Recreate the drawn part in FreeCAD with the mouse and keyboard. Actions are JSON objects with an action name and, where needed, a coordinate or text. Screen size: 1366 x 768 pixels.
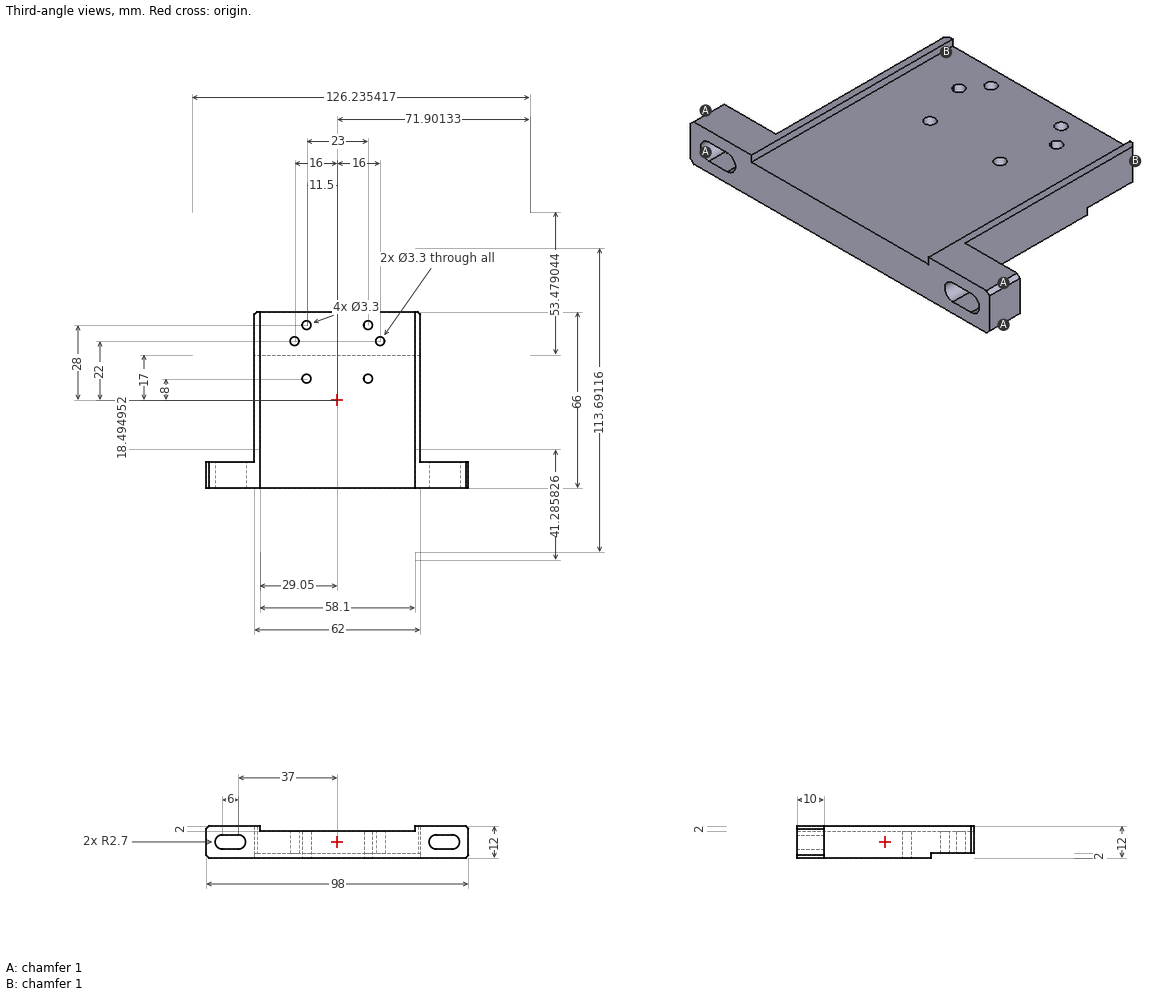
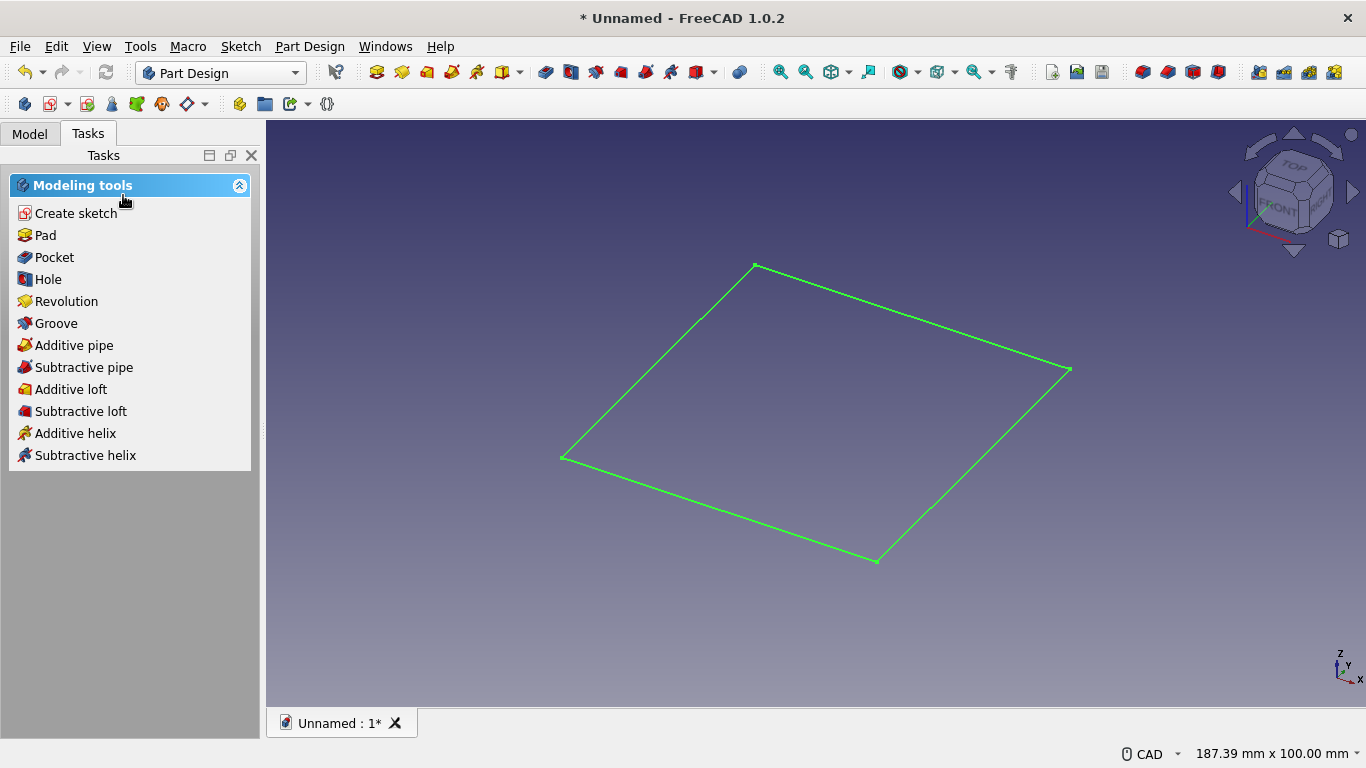
{"action": "left_click", "coordinate": [377, 72]}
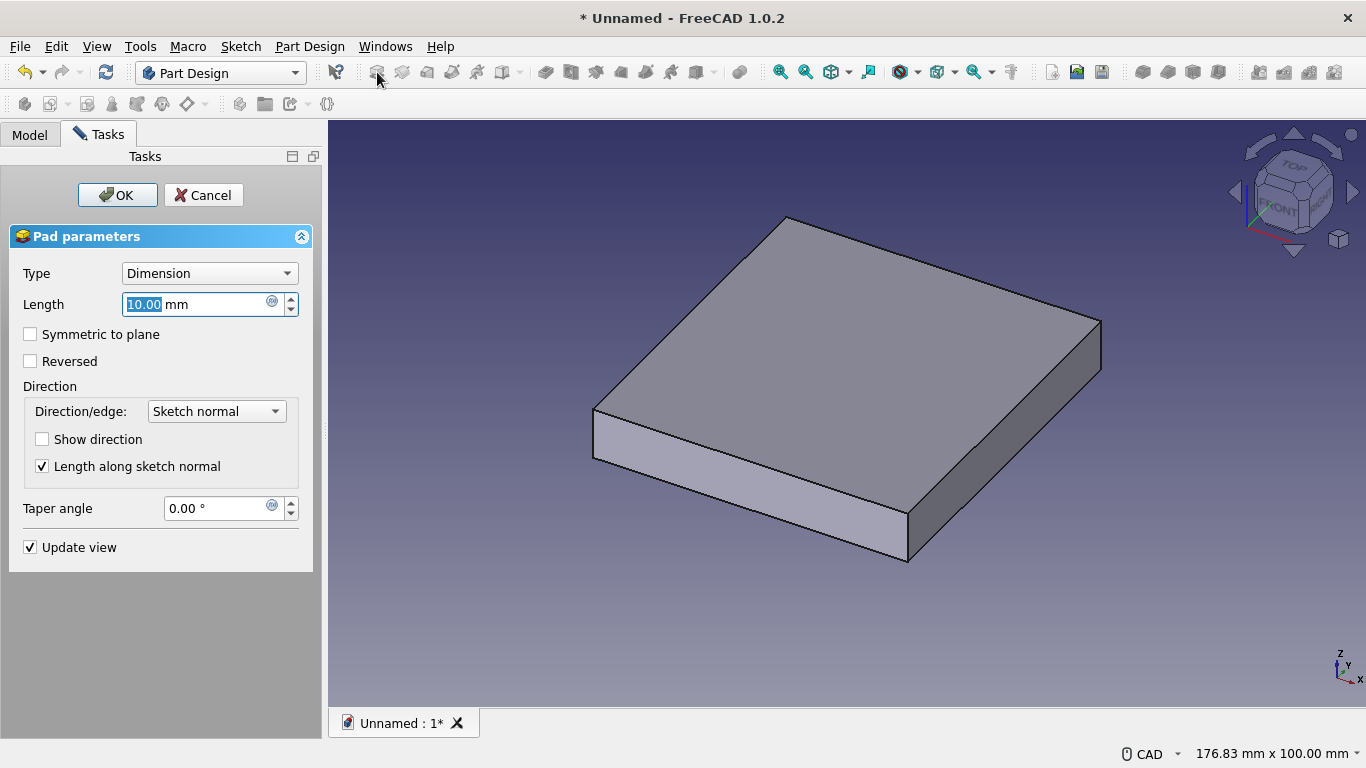
{"action": "type", "text": "12"}
{"action": "key", "text": "Tab"}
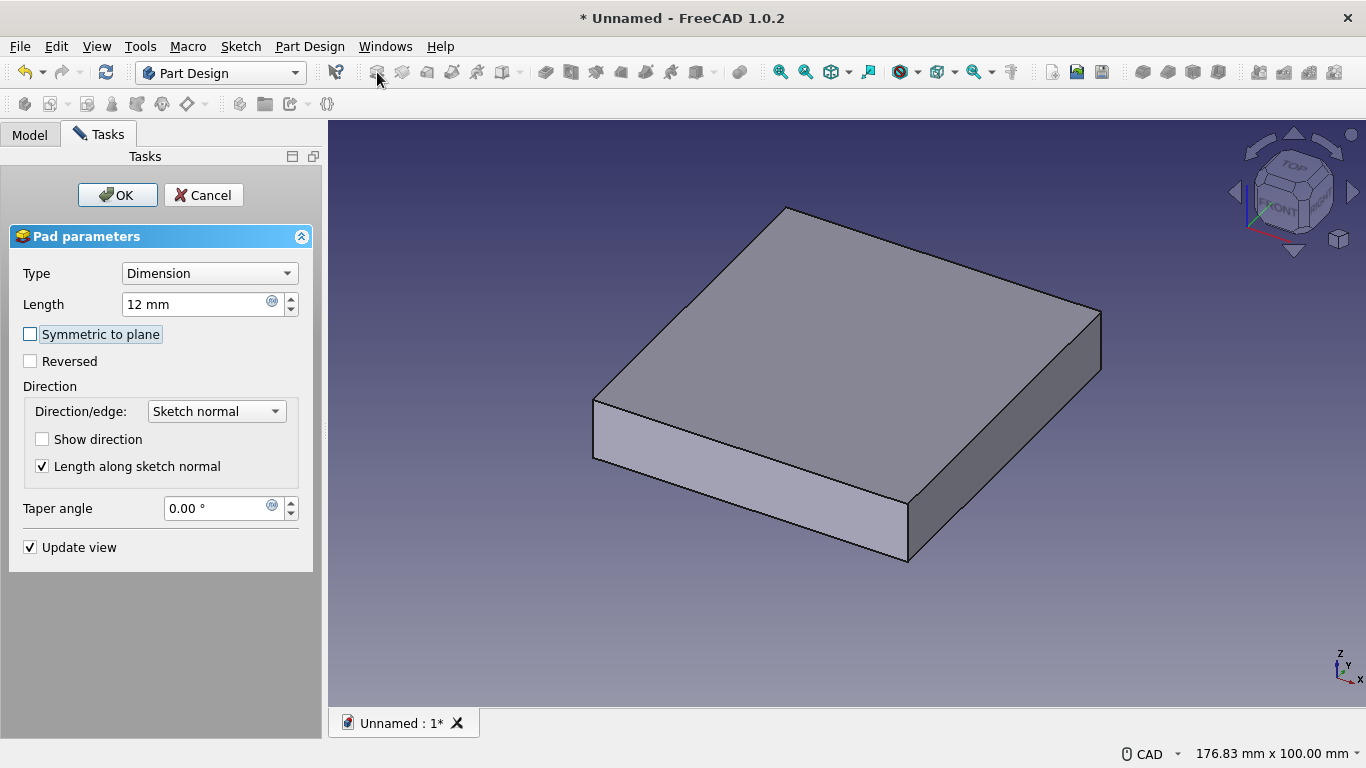
{"action": "left_click", "coordinate": [31, 334]}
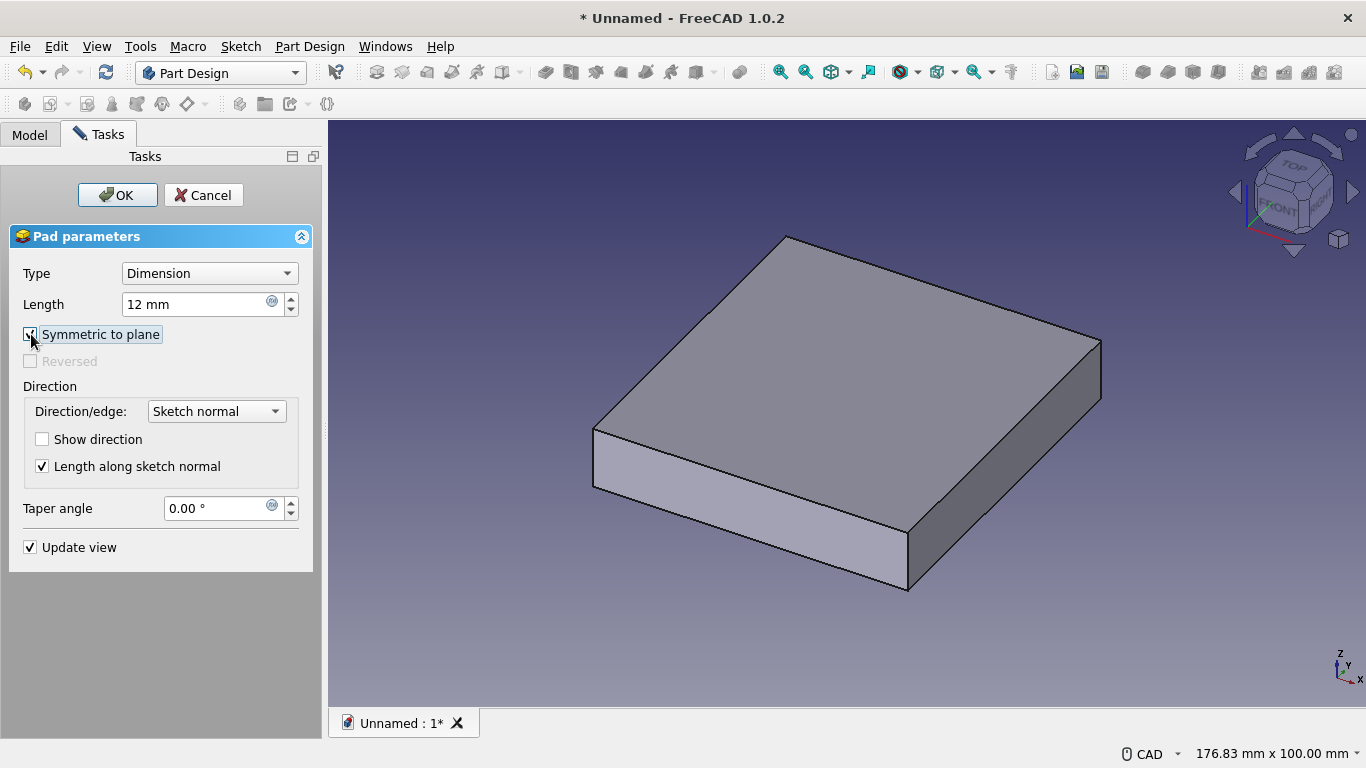
{"action": "left_click", "coordinate": [118, 195]}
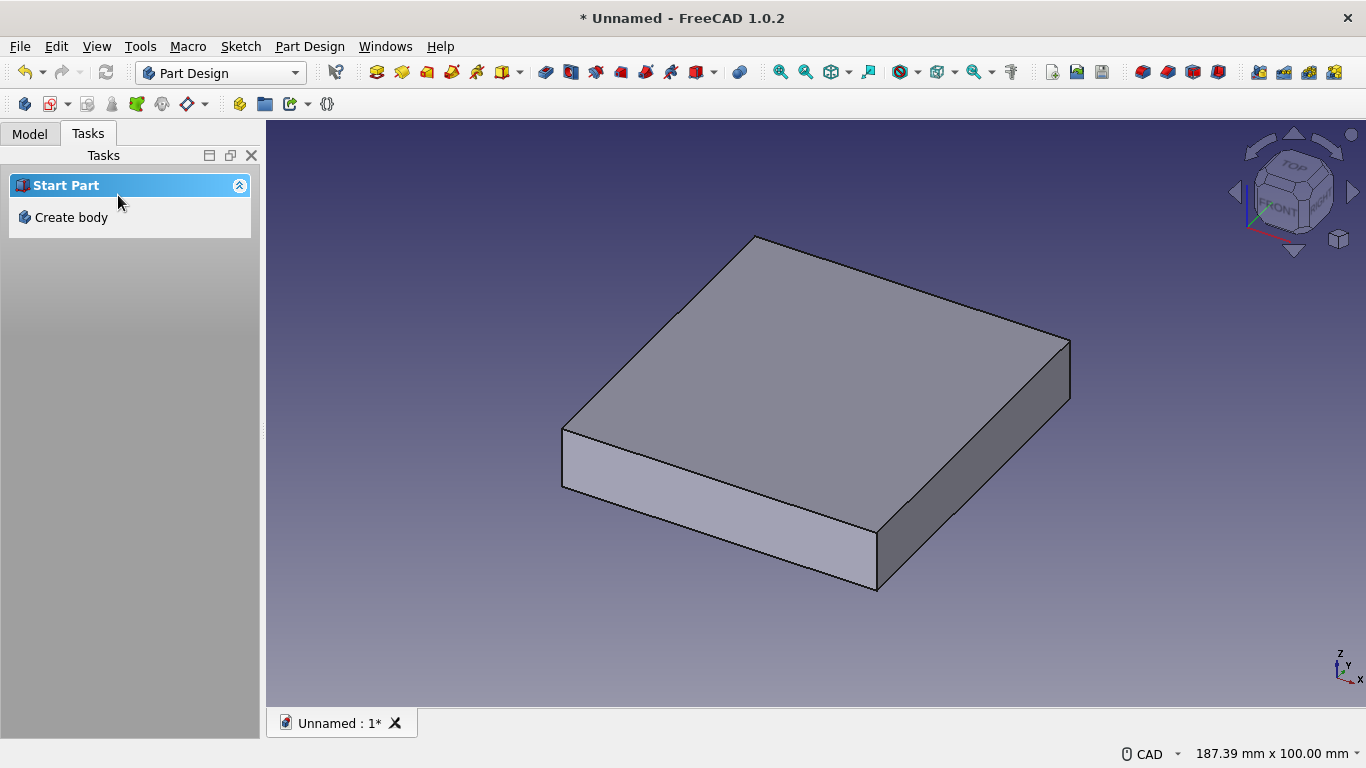
{"action": "left_click", "coordinate": [816, 384]}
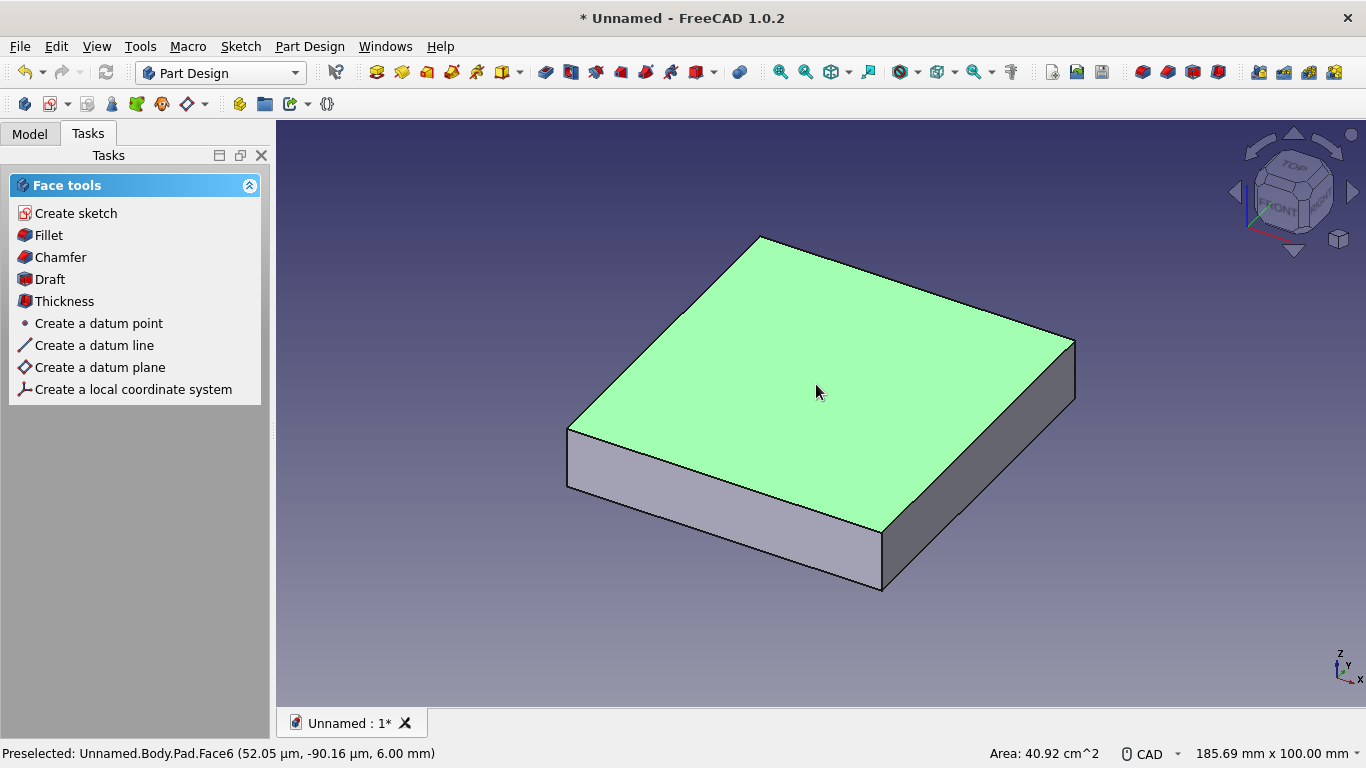
{"action": "left_click", "coordinate": [50, 104]}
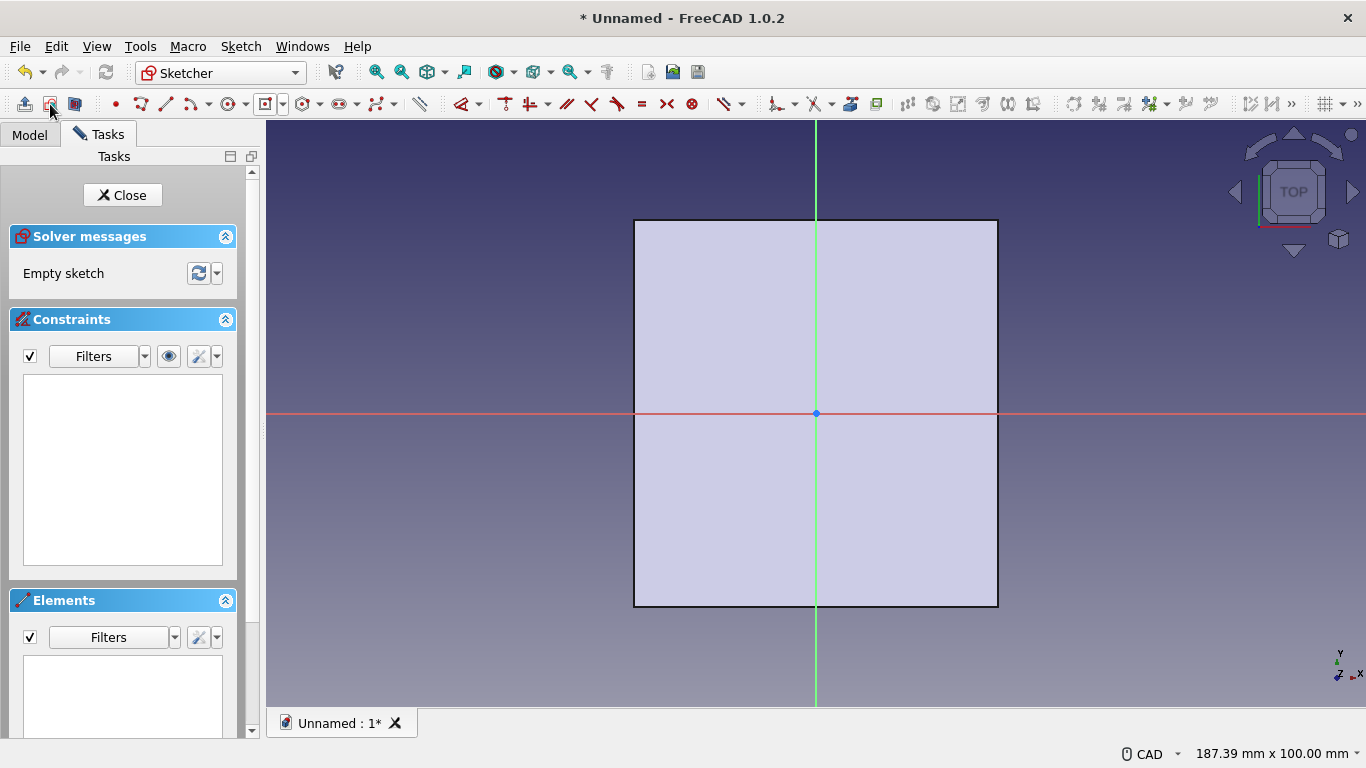
{"action": "scroll", "coordinate": [664, 414], "scroll_direction": "down", "scroll_amount": 3}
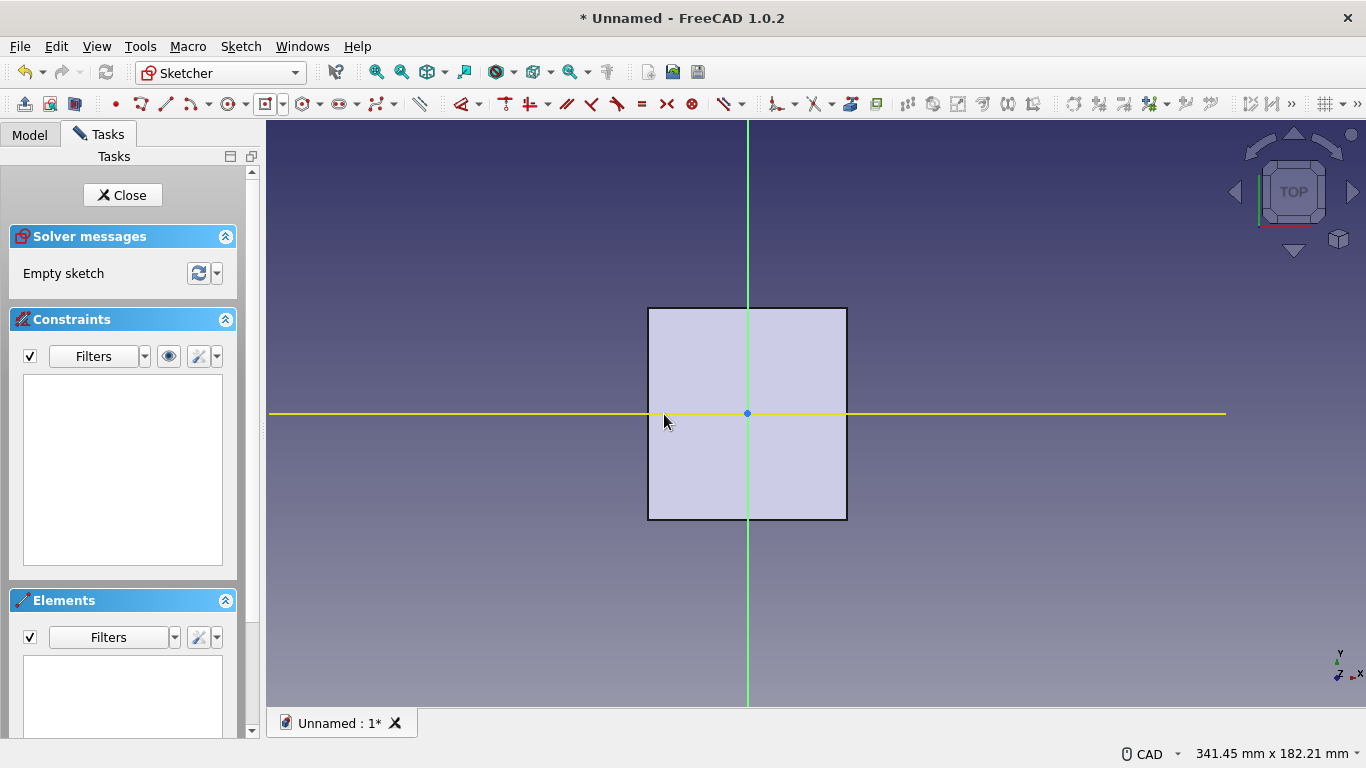
{"action": "left_click", "coordinate": [264, 104]}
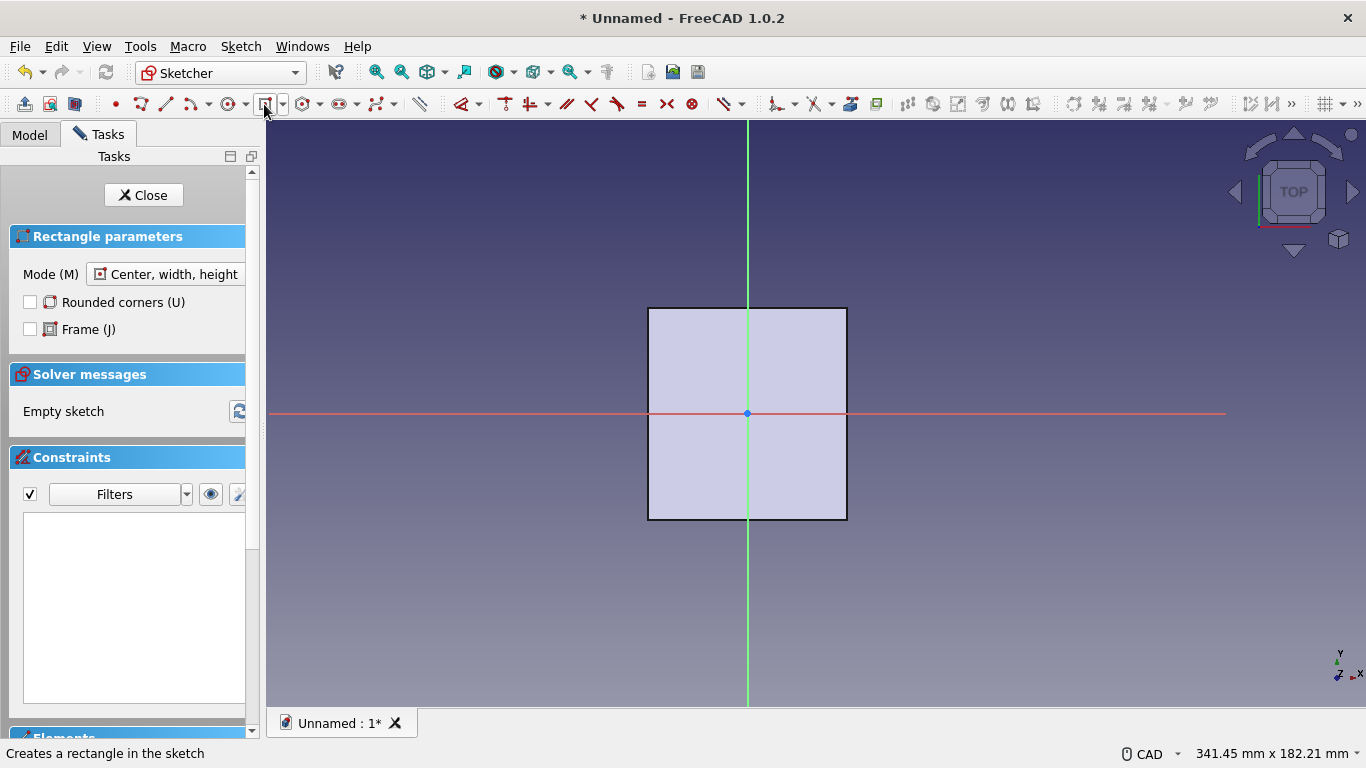
{"action": "left_click", "coordinate": [748, 414]}
{"action": "mouse_move", "coordinate": [841, 231]}